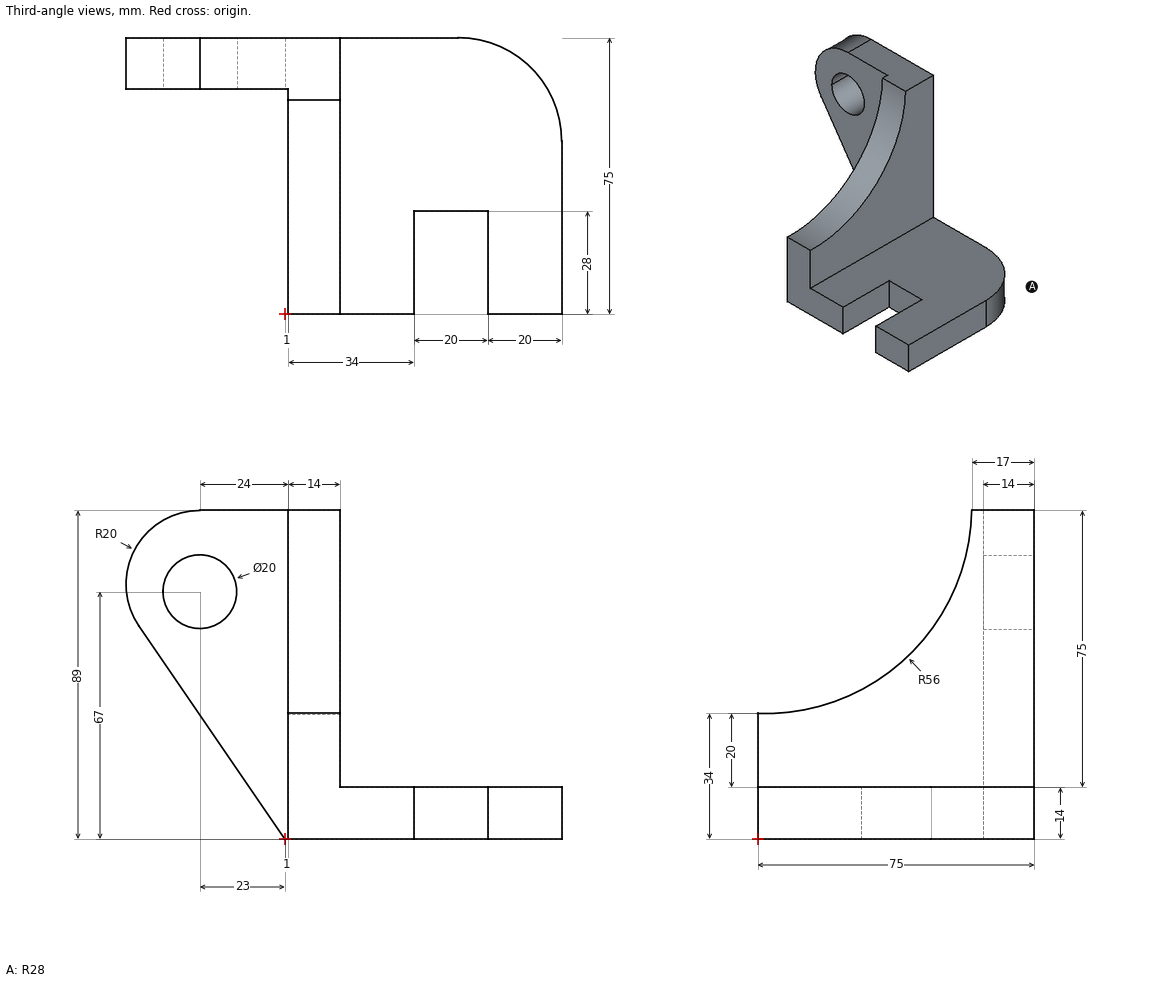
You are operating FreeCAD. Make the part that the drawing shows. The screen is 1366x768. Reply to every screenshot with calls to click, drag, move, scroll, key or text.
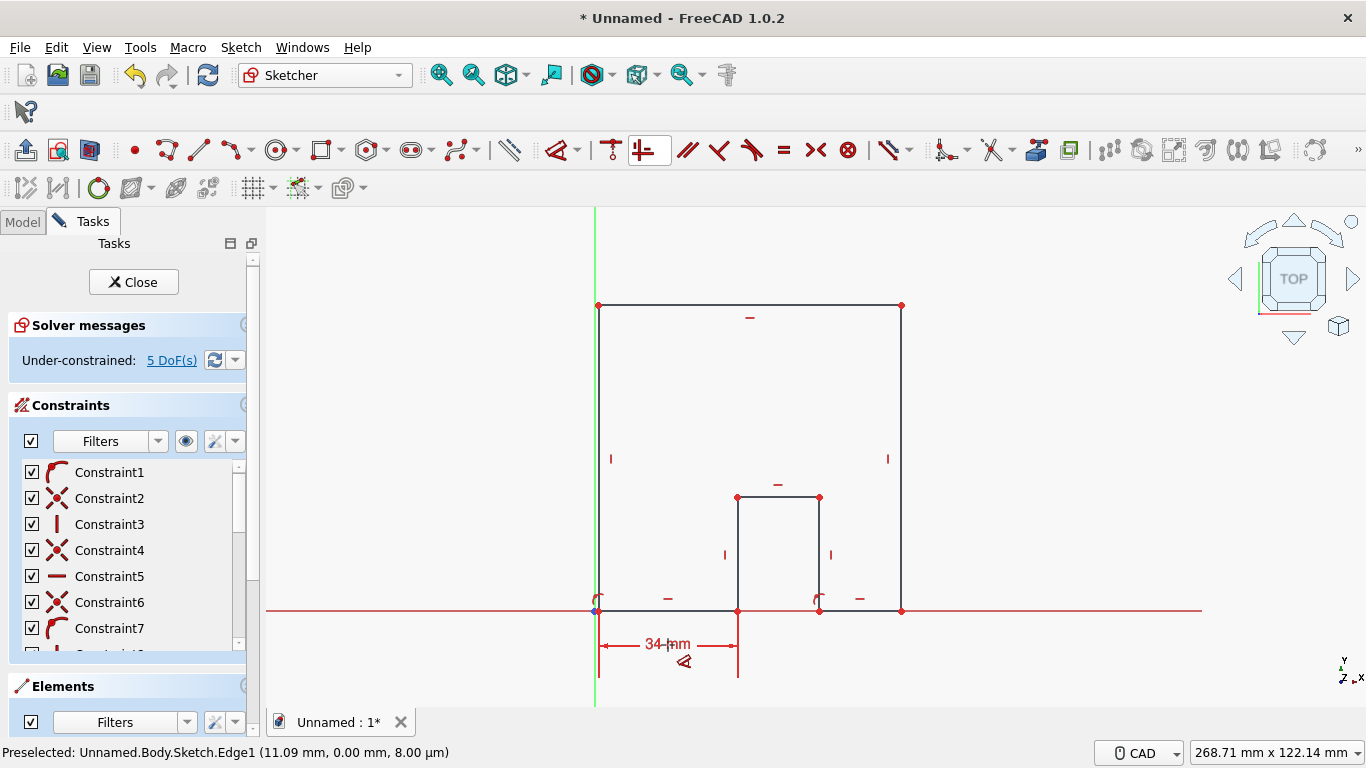
click(738, 577)
click(704, 554)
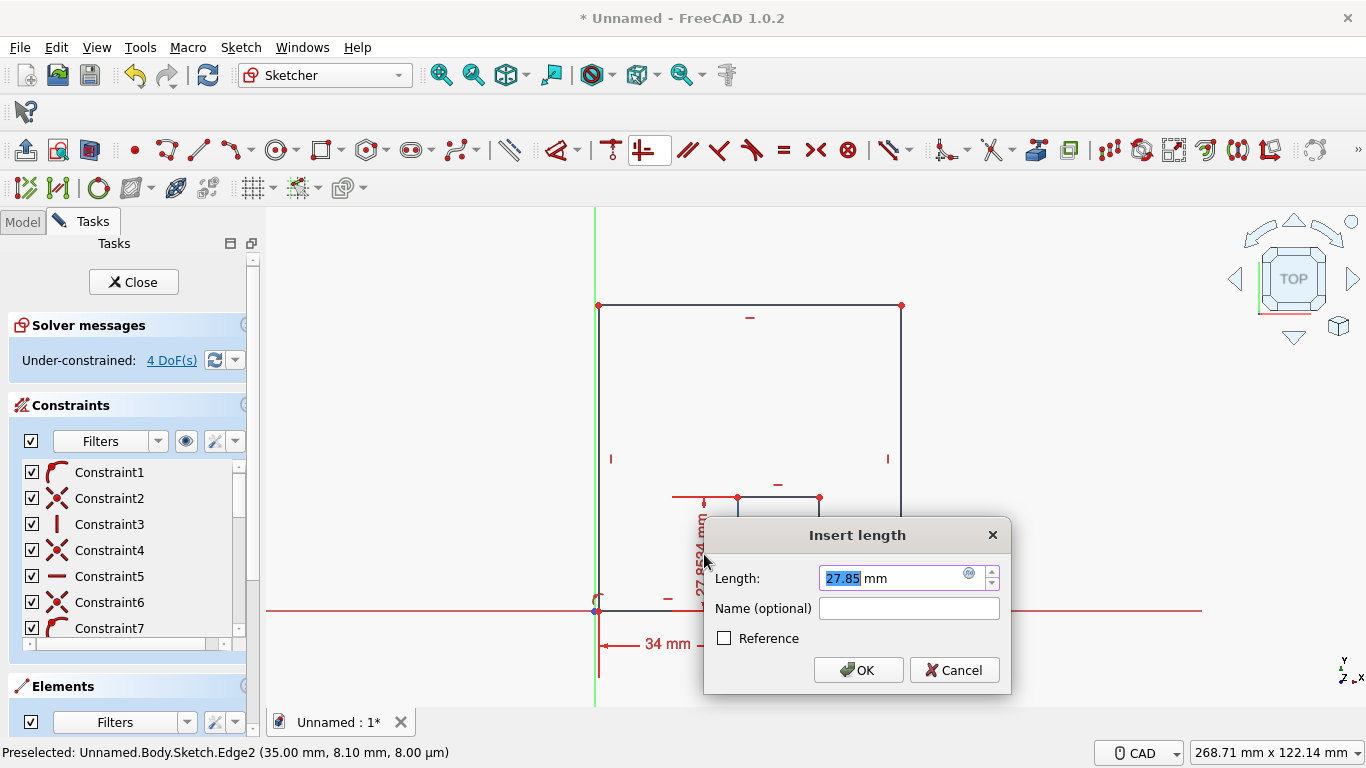
text(28)
key(Return)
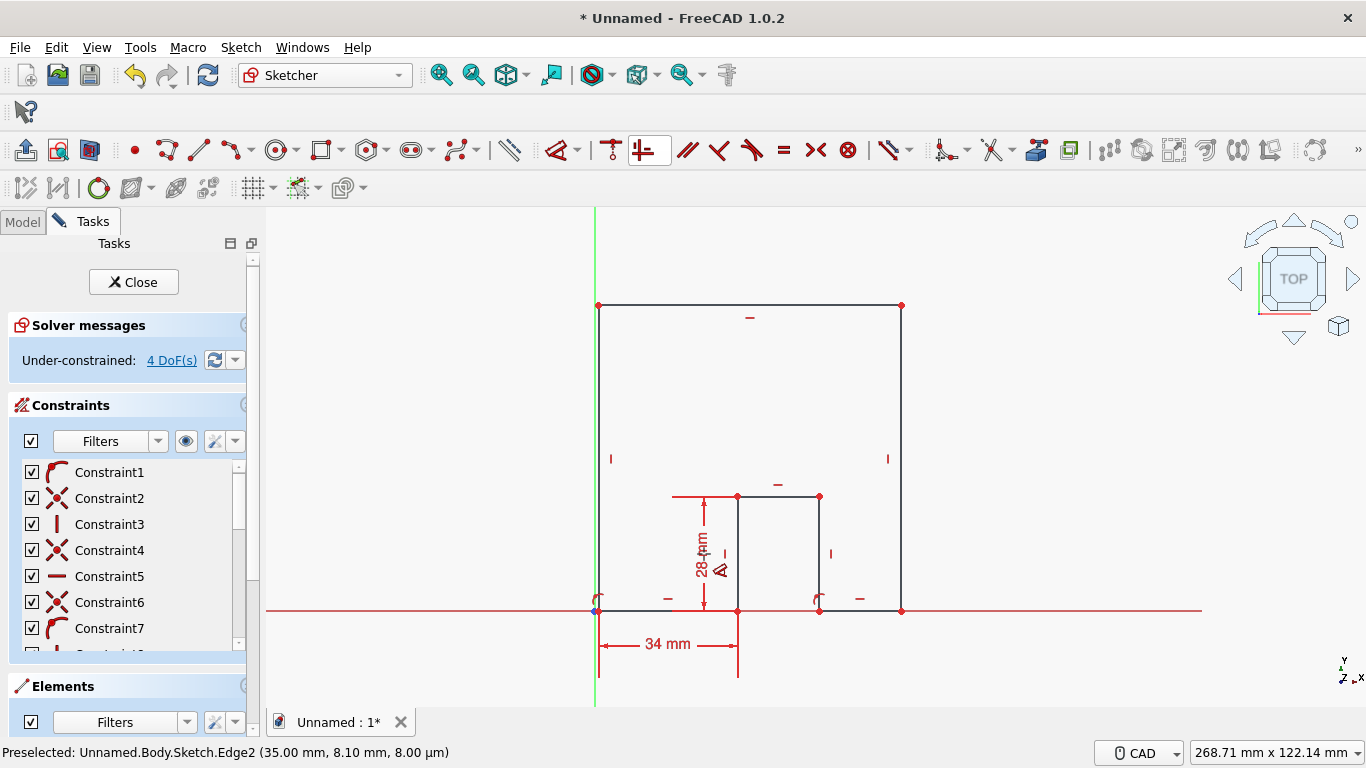
click(762, 497)
click(779, 531)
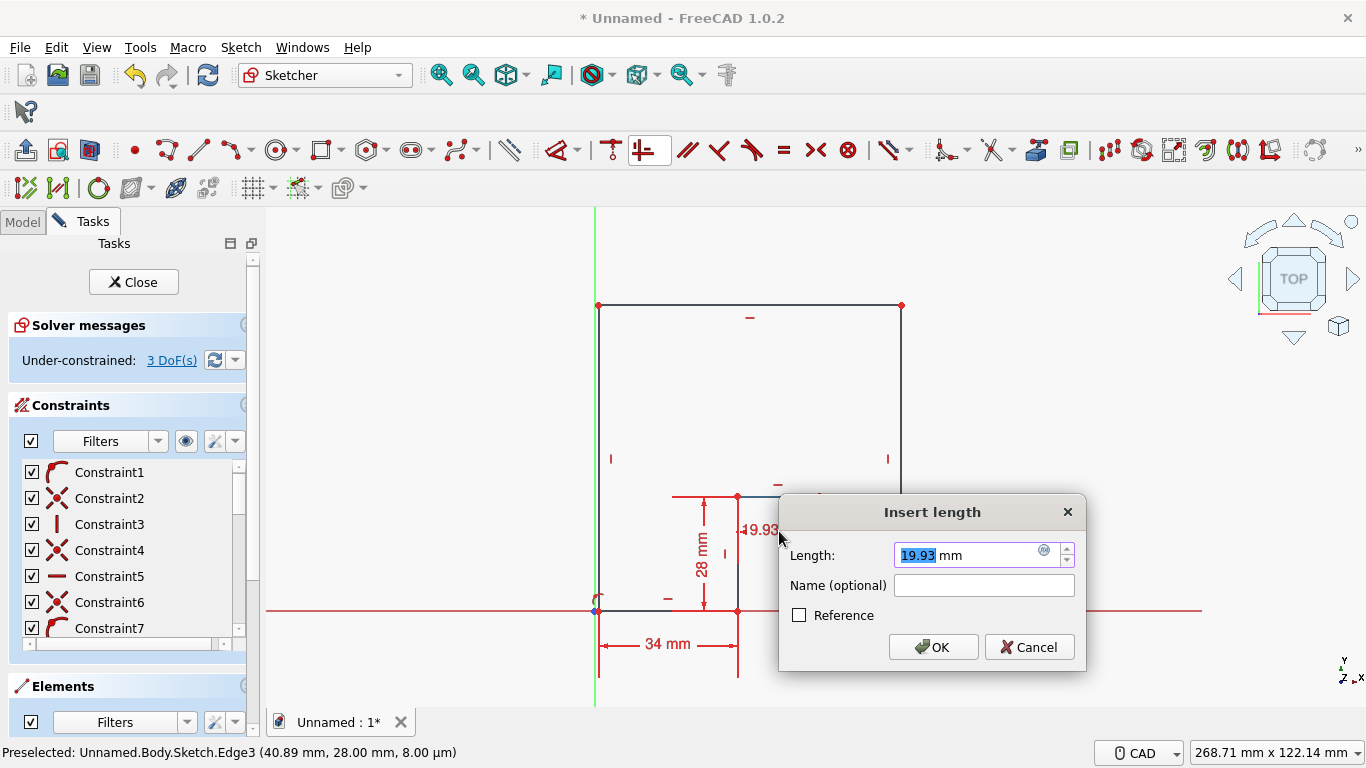
text(20)
key(Return)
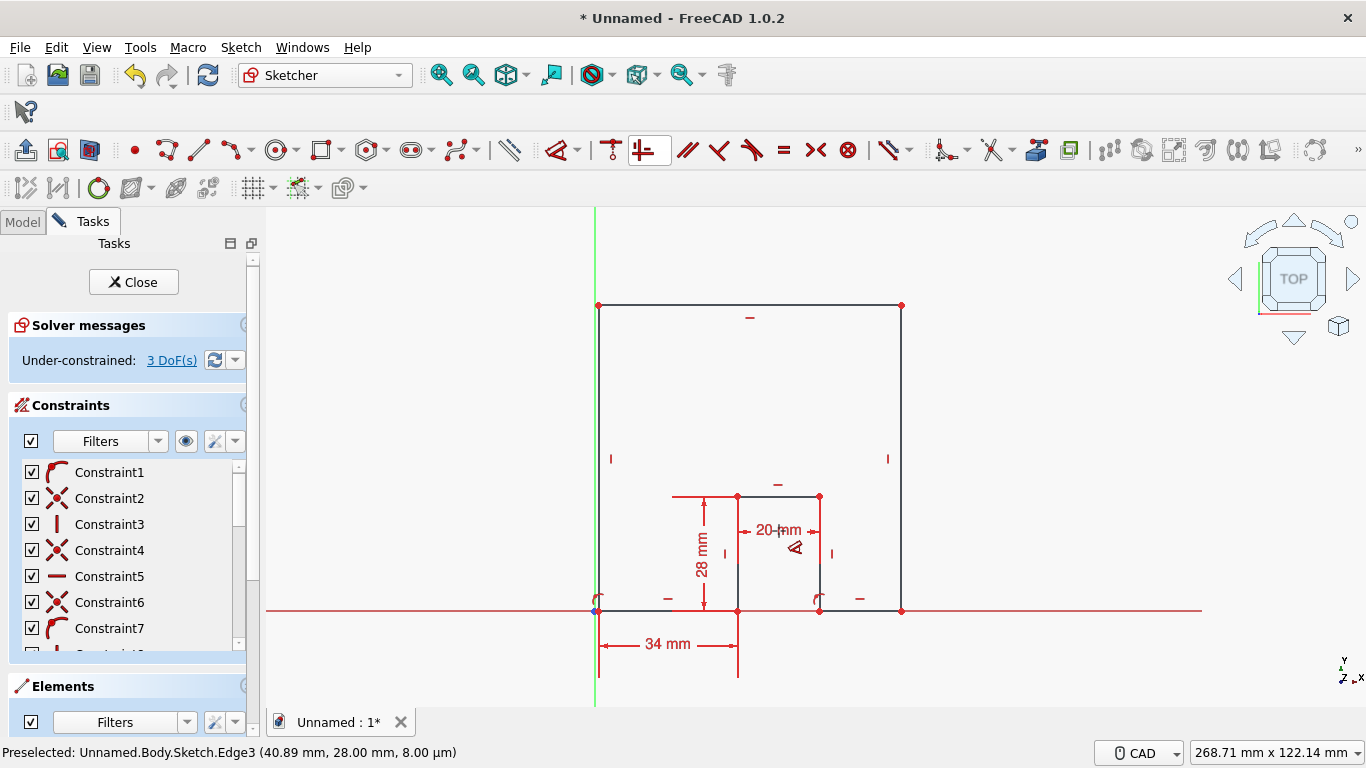
click(844, 611)
click(861, 645)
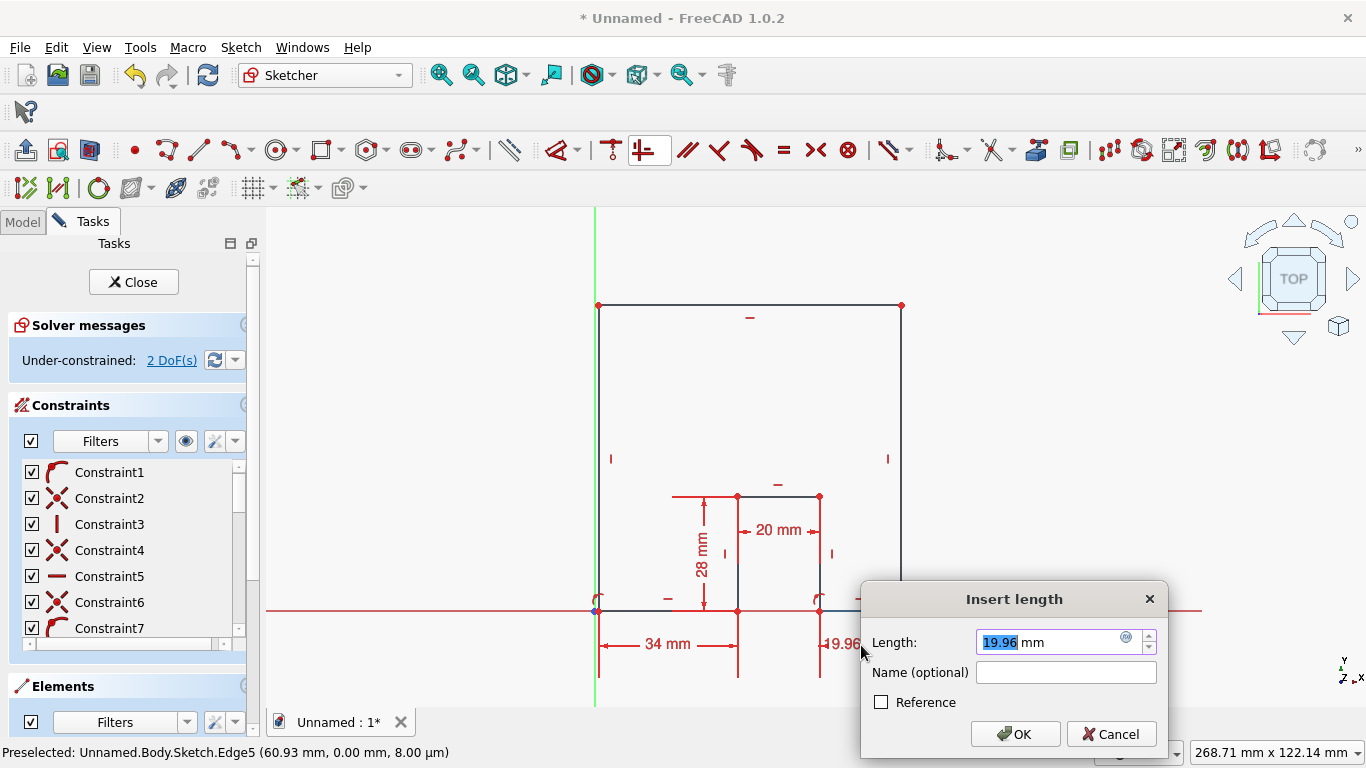
text(20)
key(Return)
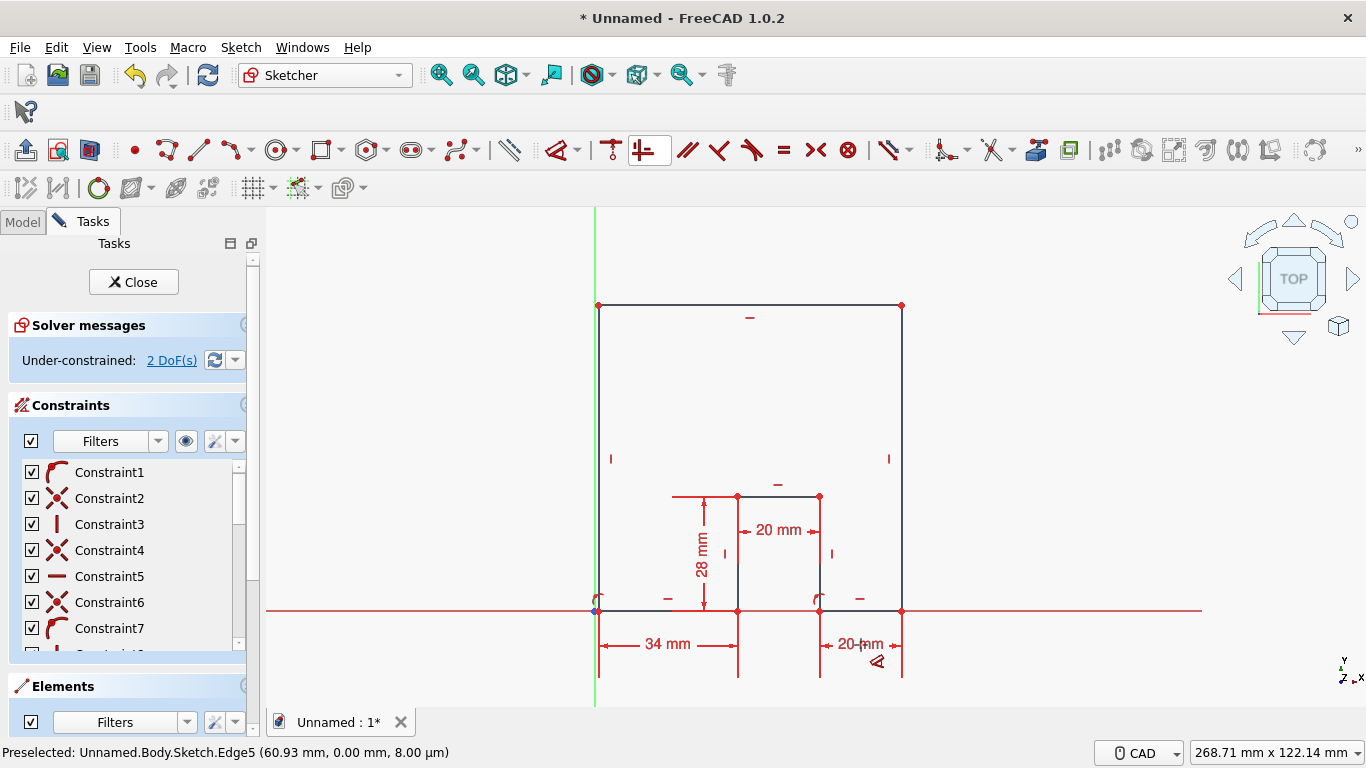
click(902, 519)
click(936, 458)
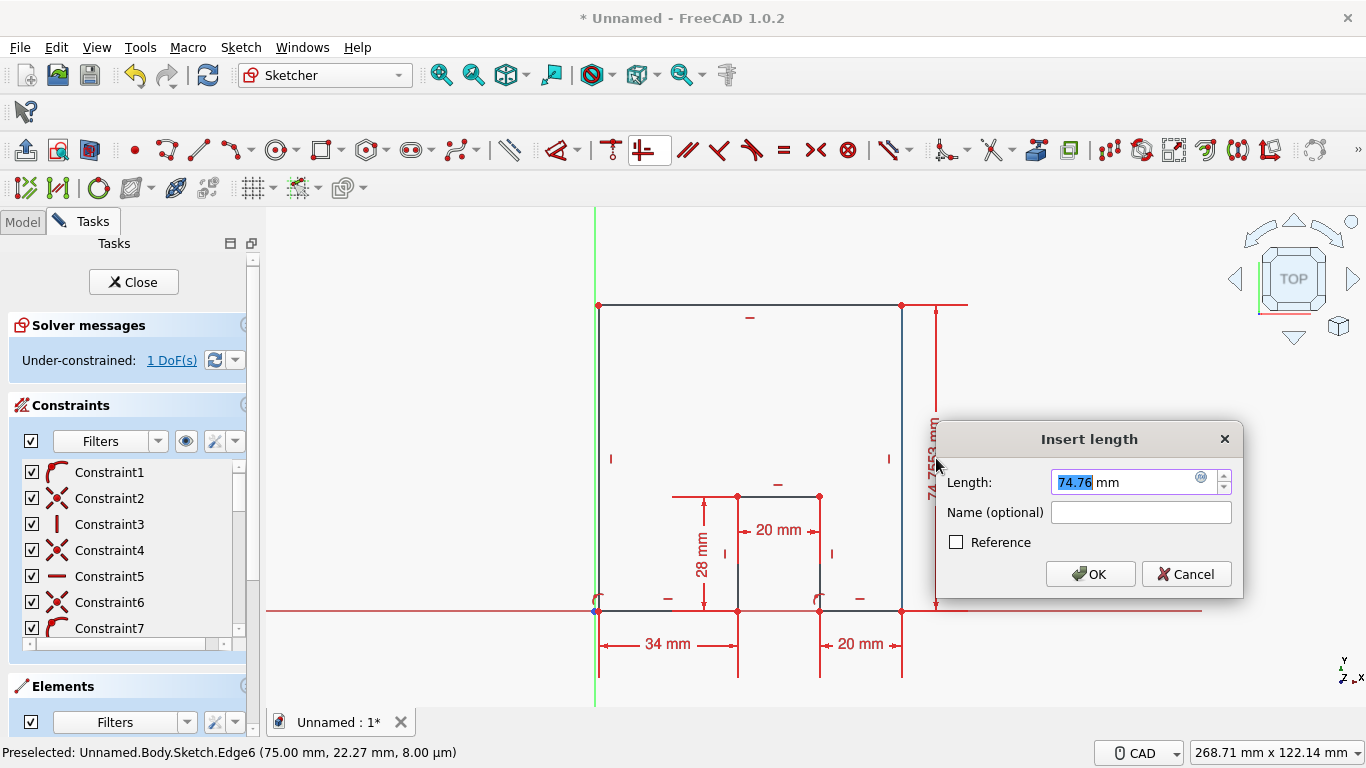
text(75)
key(Return)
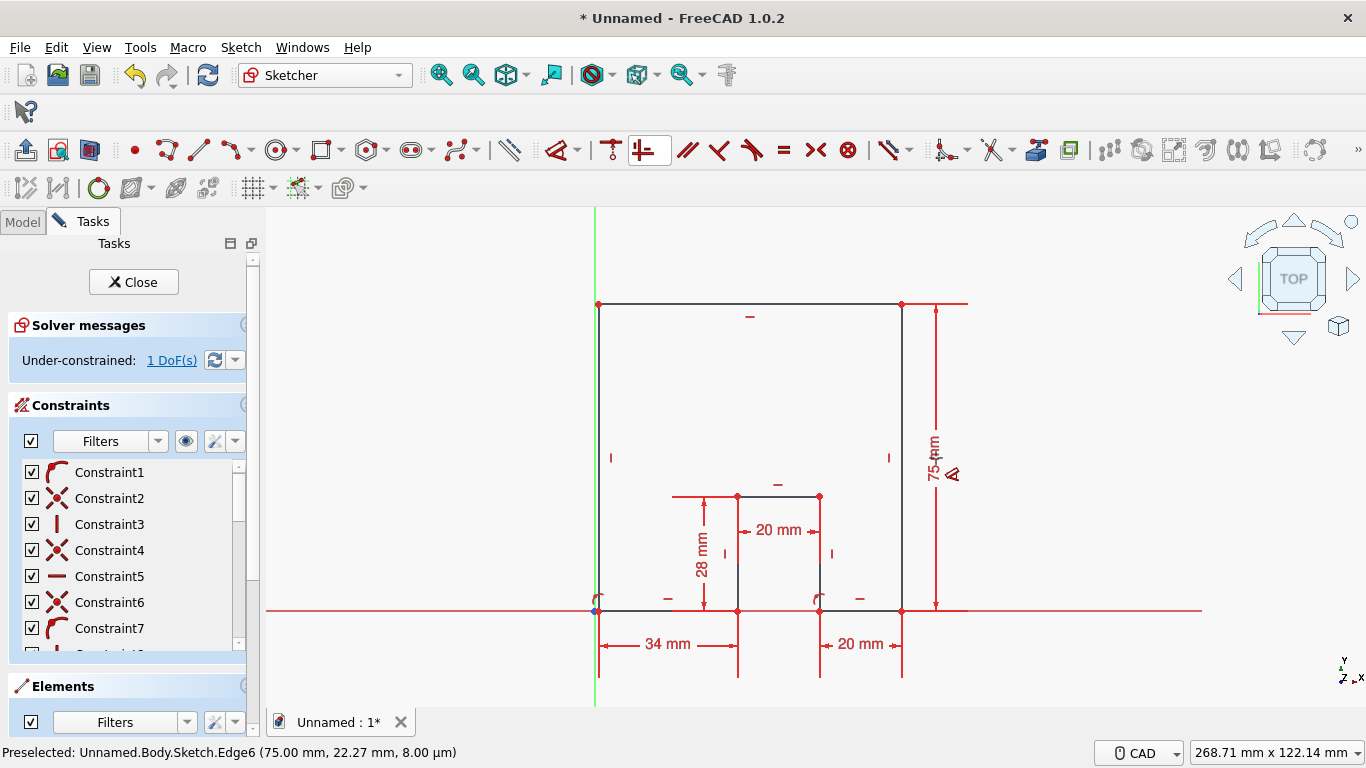
scroll(599, 611, up, 12)